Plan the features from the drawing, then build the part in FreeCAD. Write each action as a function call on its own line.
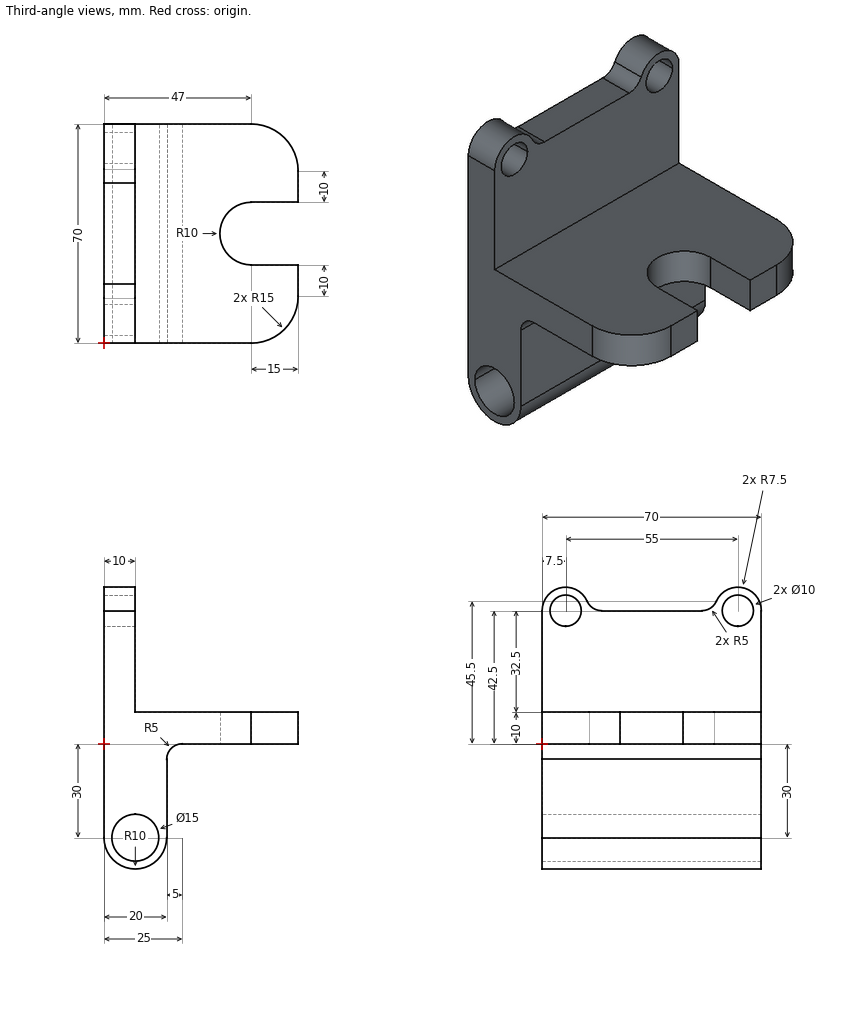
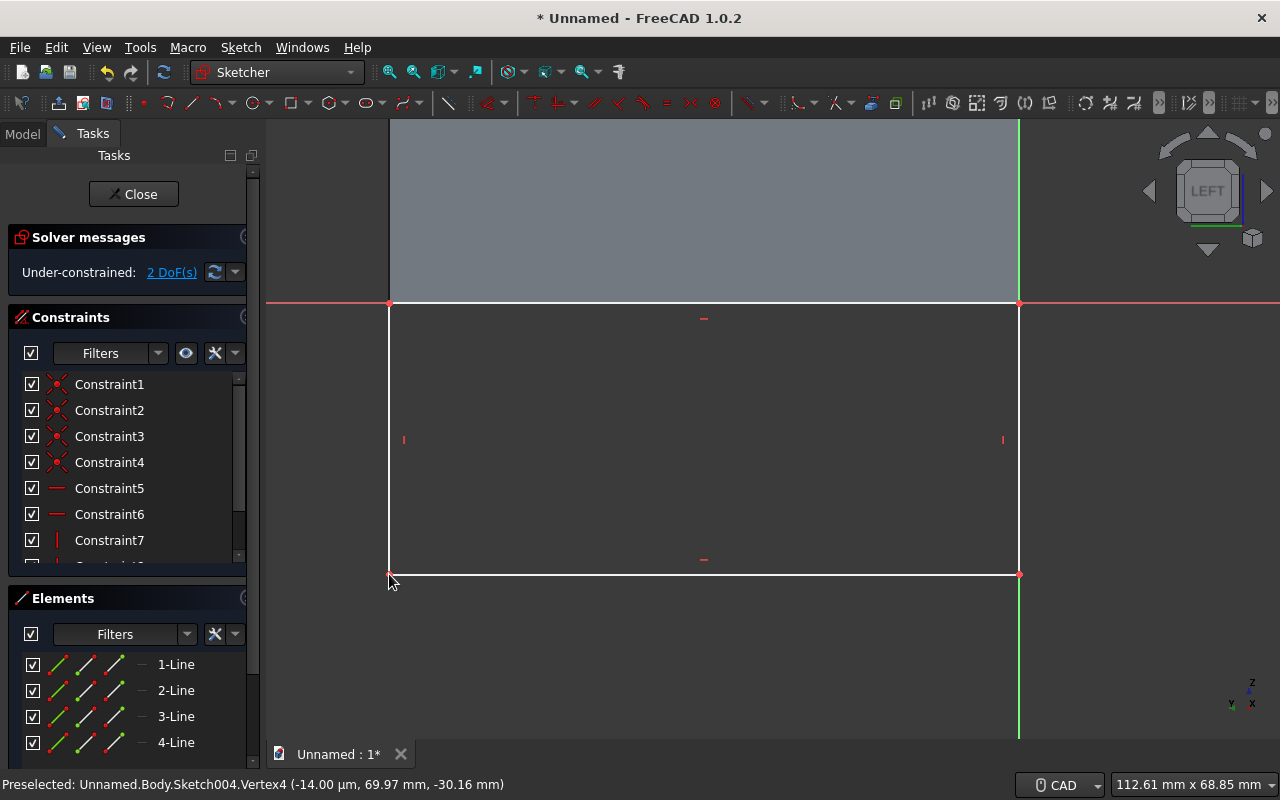
click(488, 104)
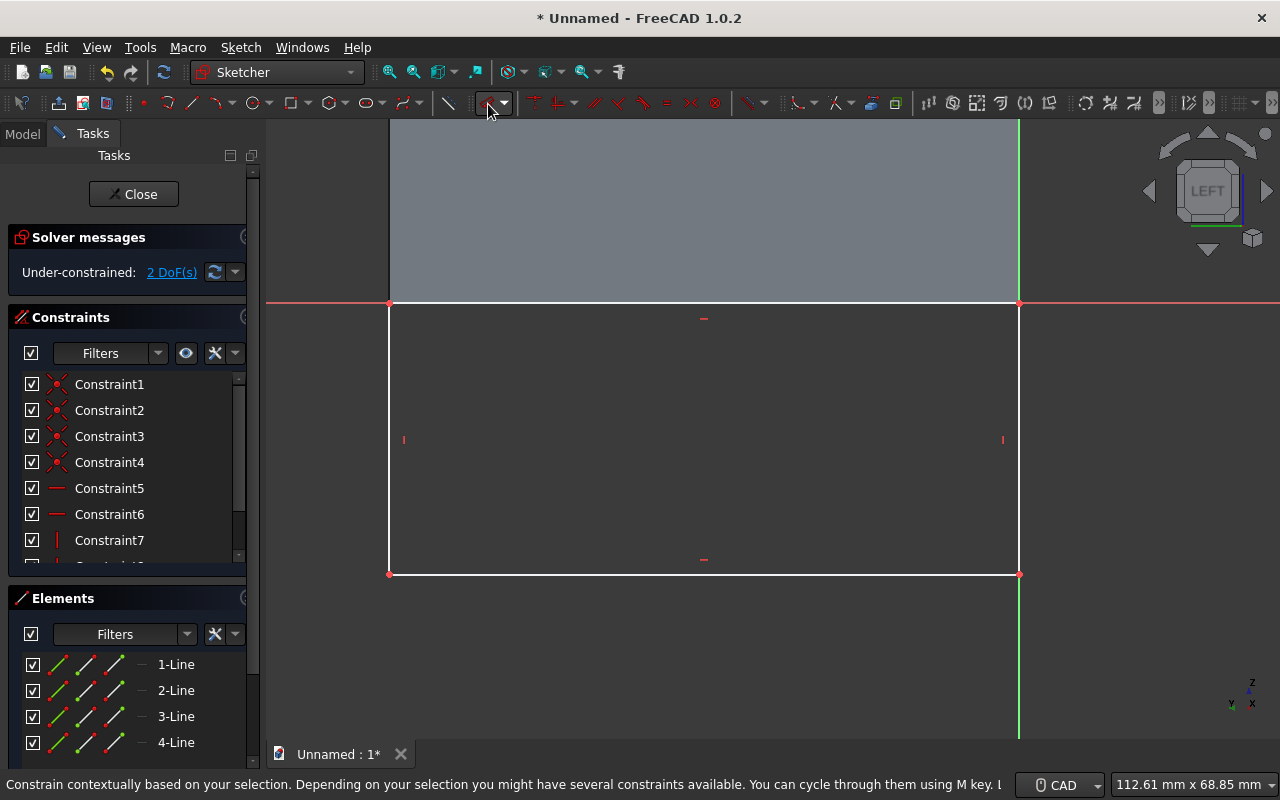
click(830, 303)
click(704, 269)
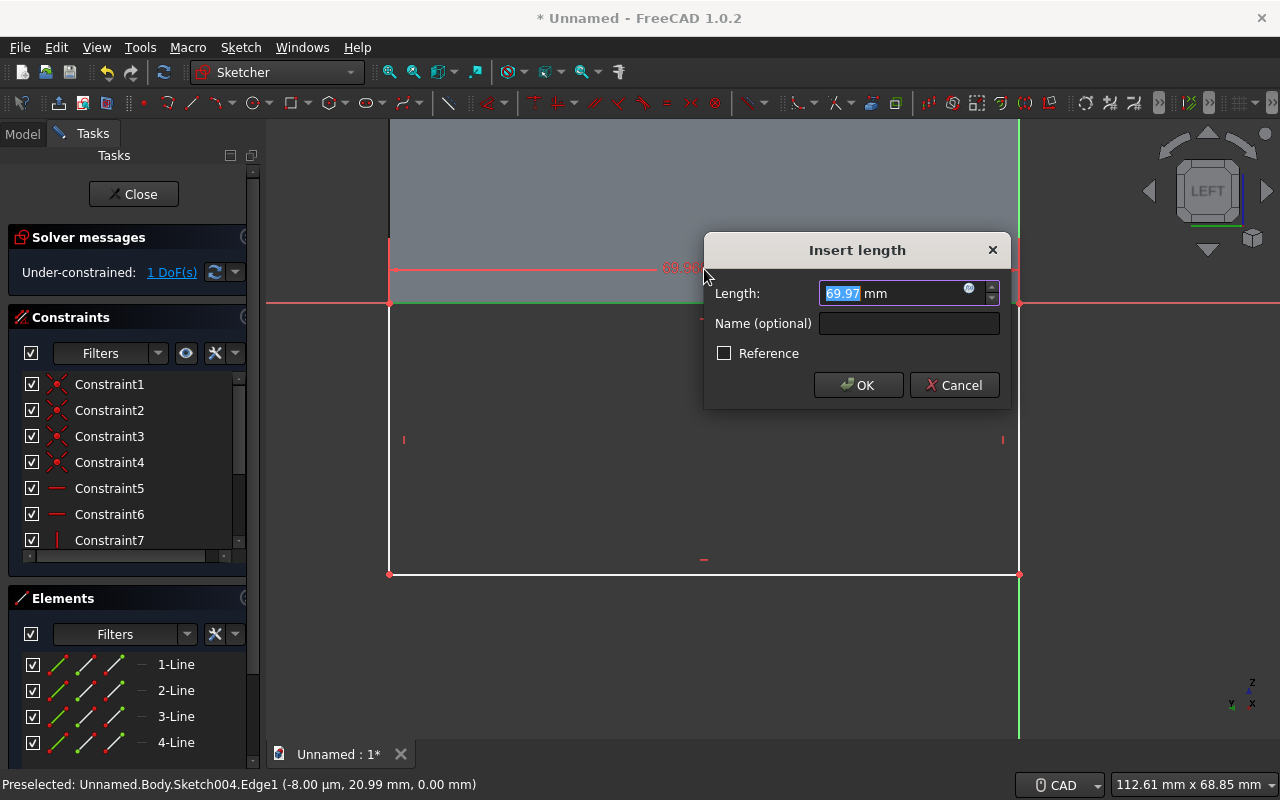
text(70)
key(Return)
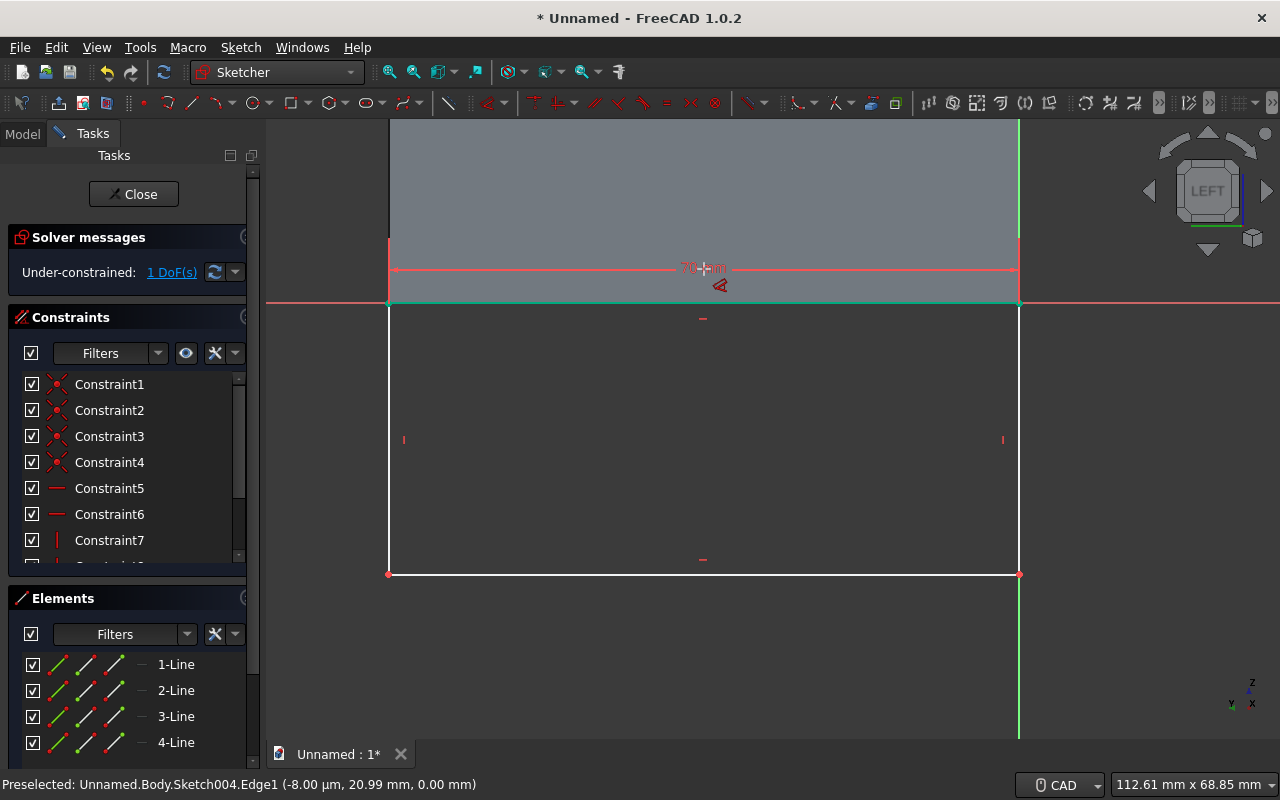
click(389, 385)
click(355, 439)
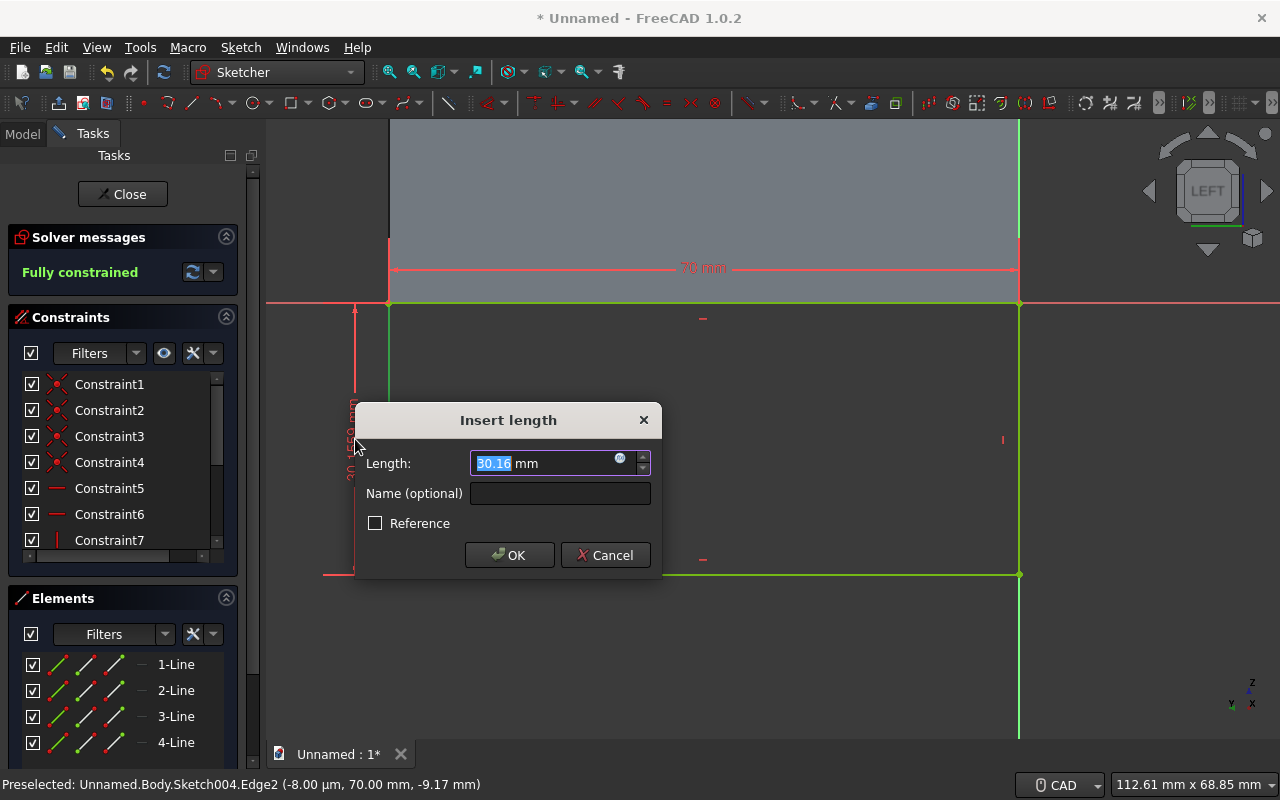
text(30)
key(Return)
key(Escape)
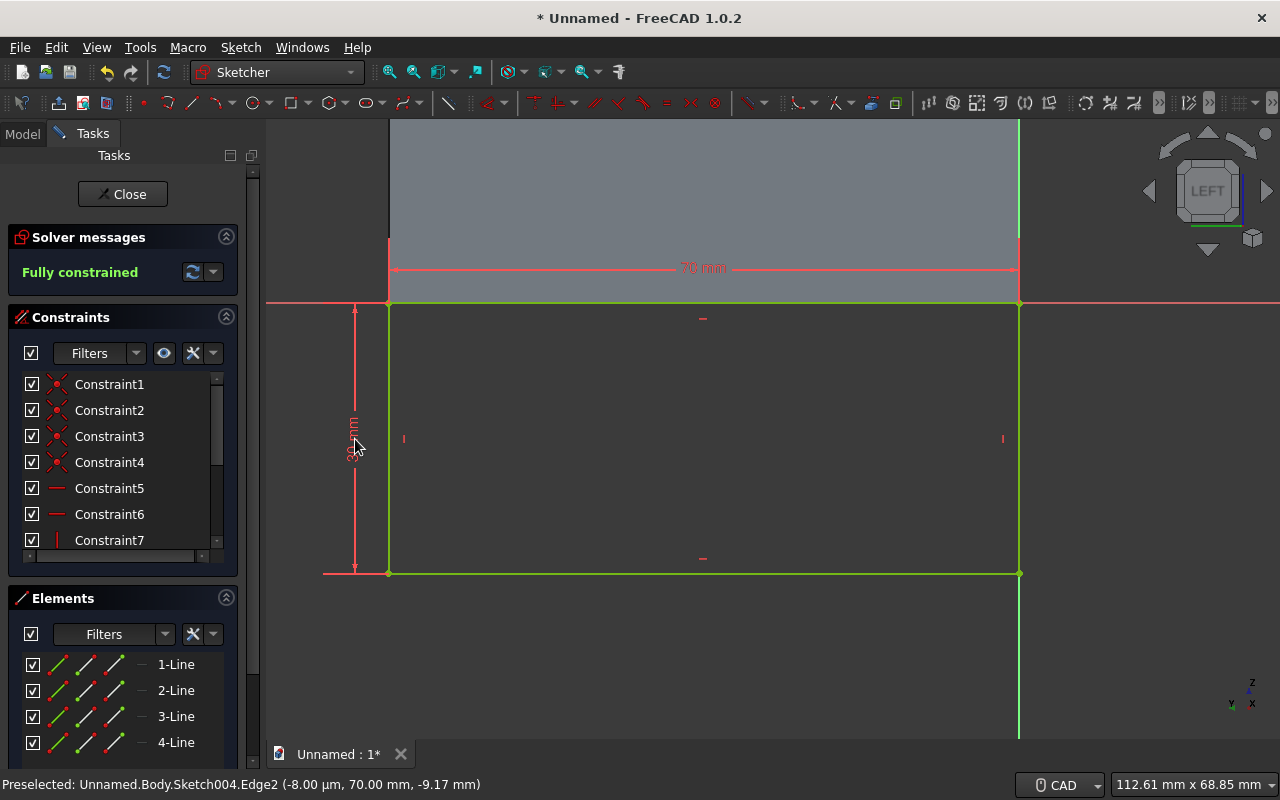
click(123, 194)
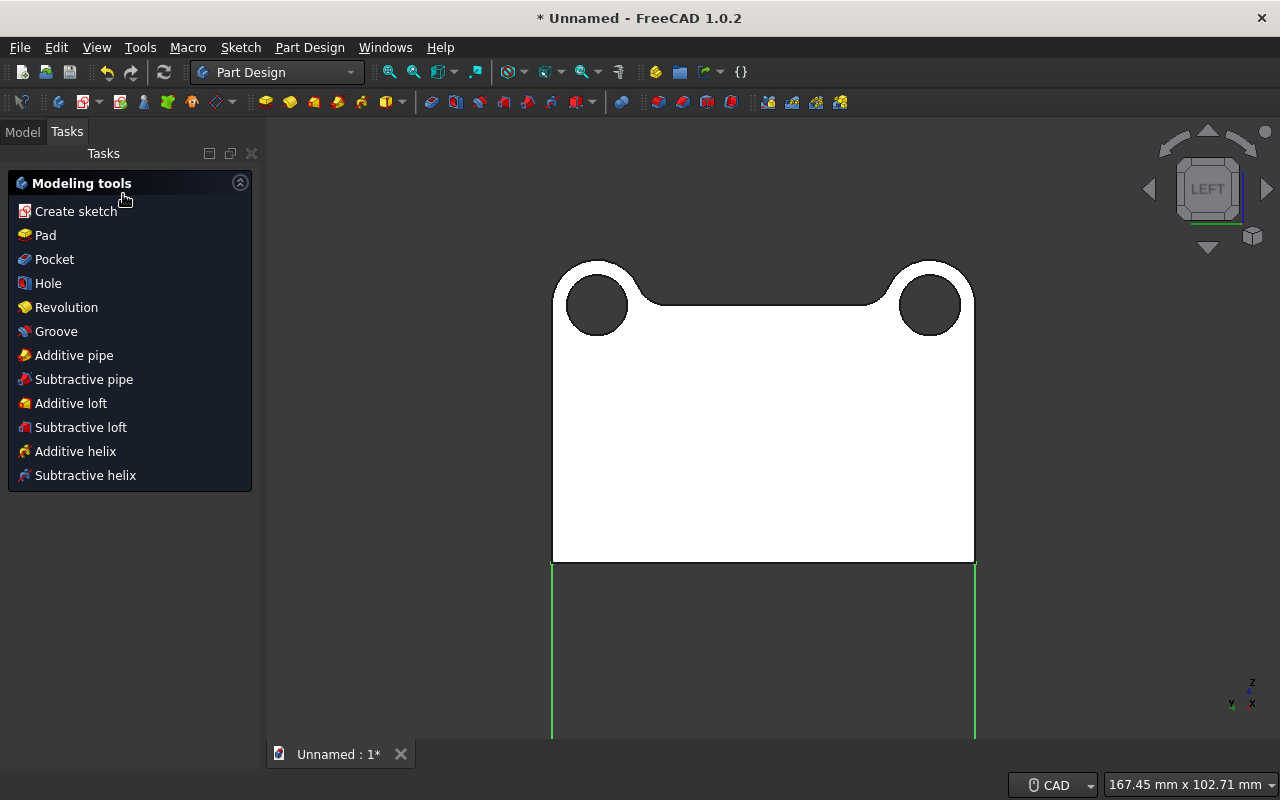
click(266, 102)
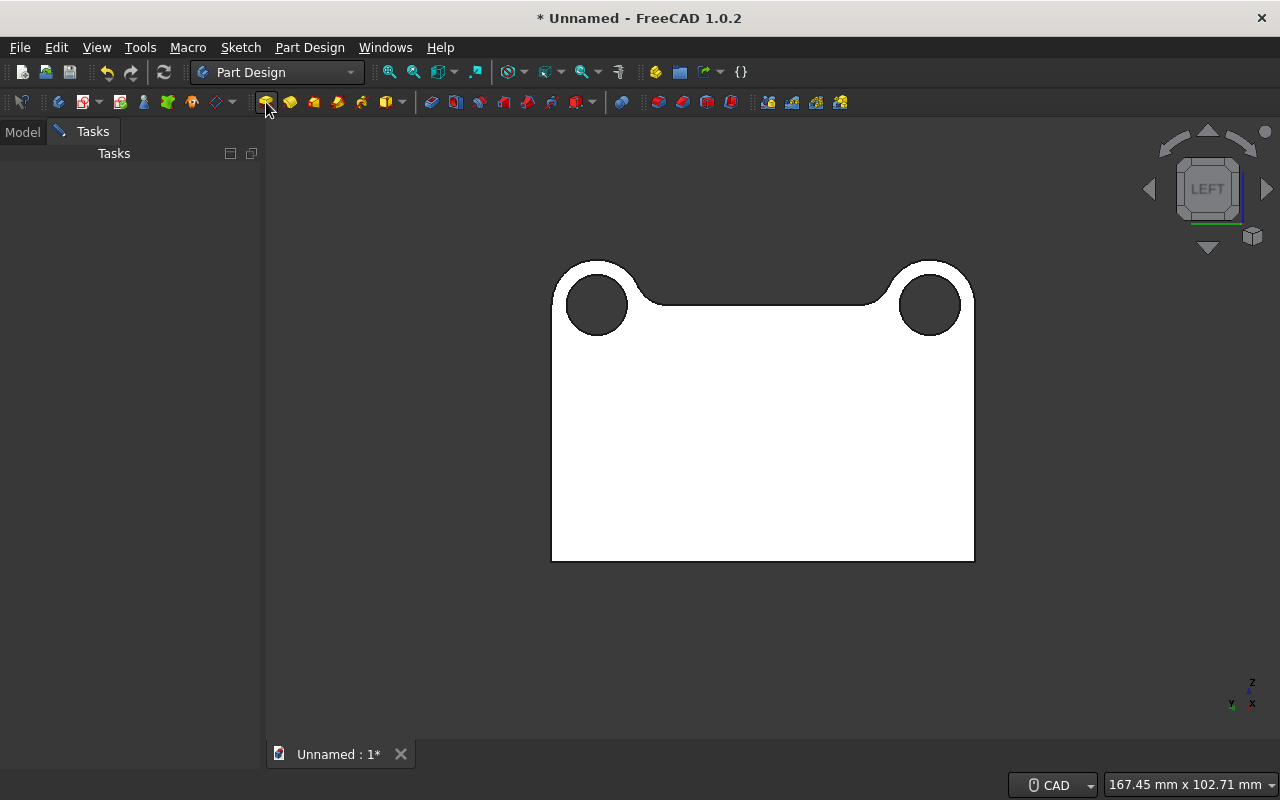
text(25)
key(Tab)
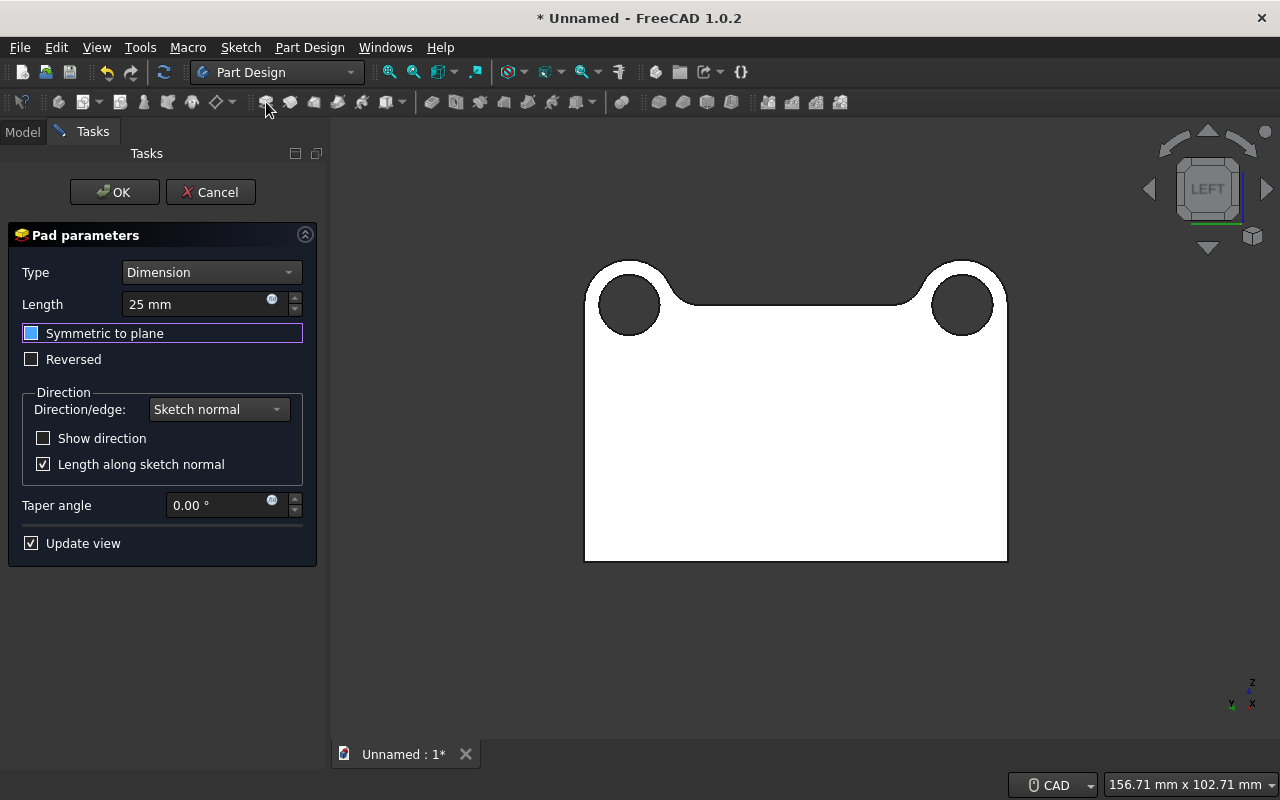
click(30, 359)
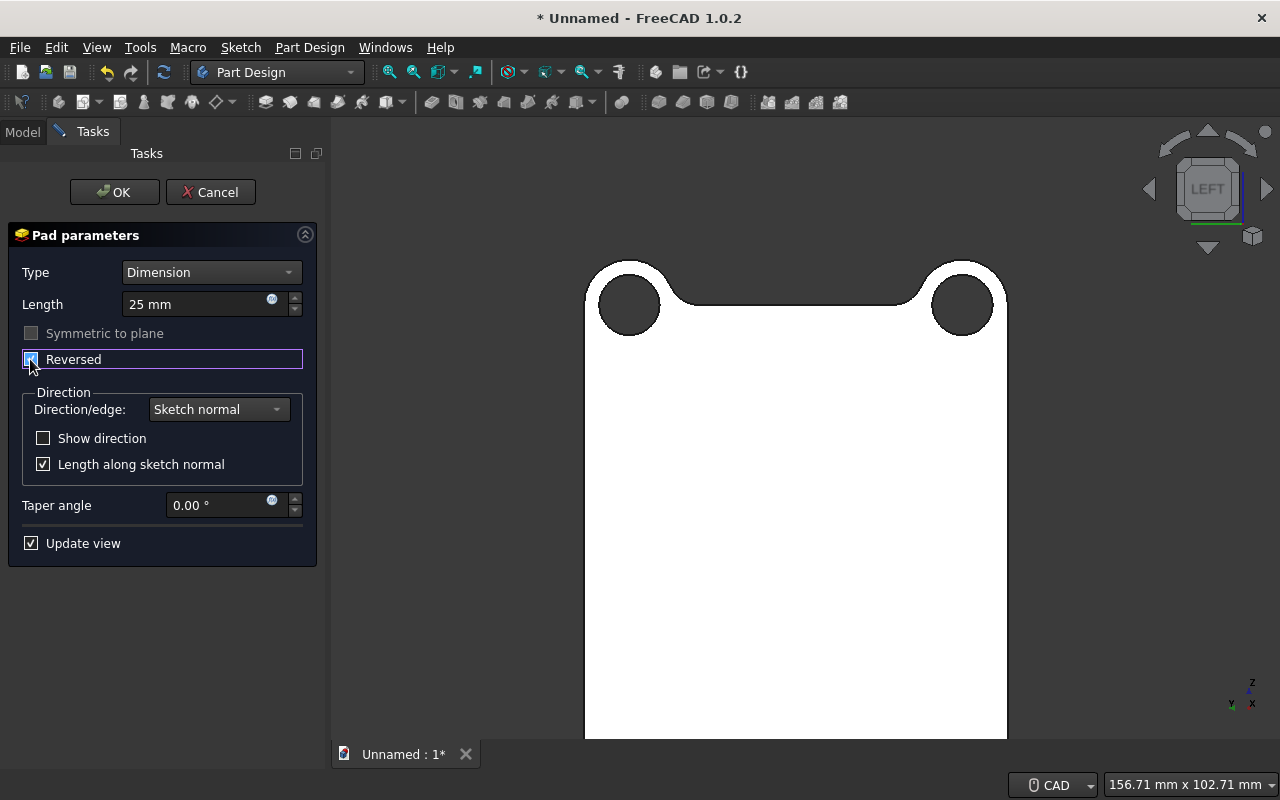
click(115, 192)